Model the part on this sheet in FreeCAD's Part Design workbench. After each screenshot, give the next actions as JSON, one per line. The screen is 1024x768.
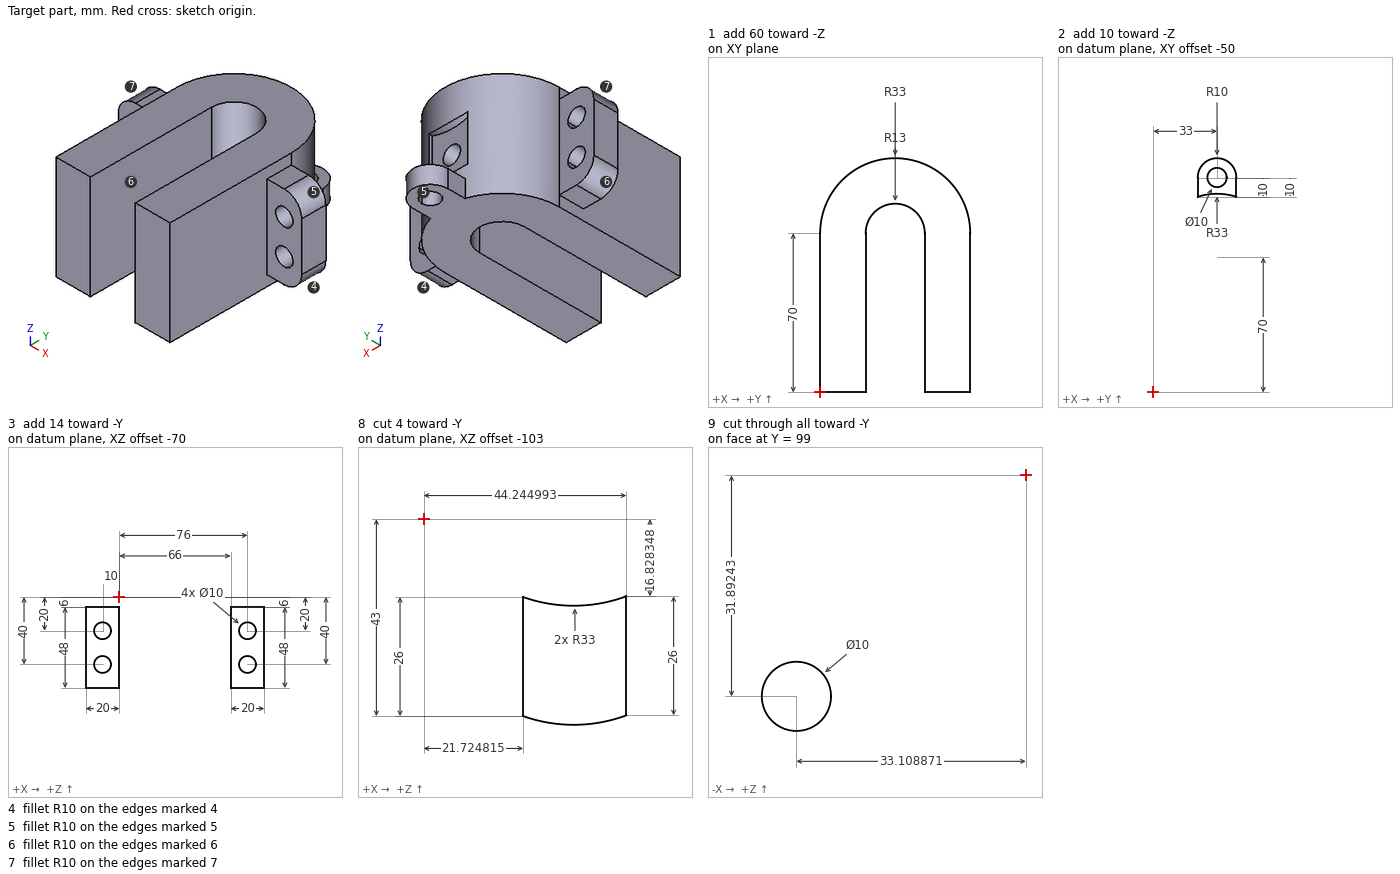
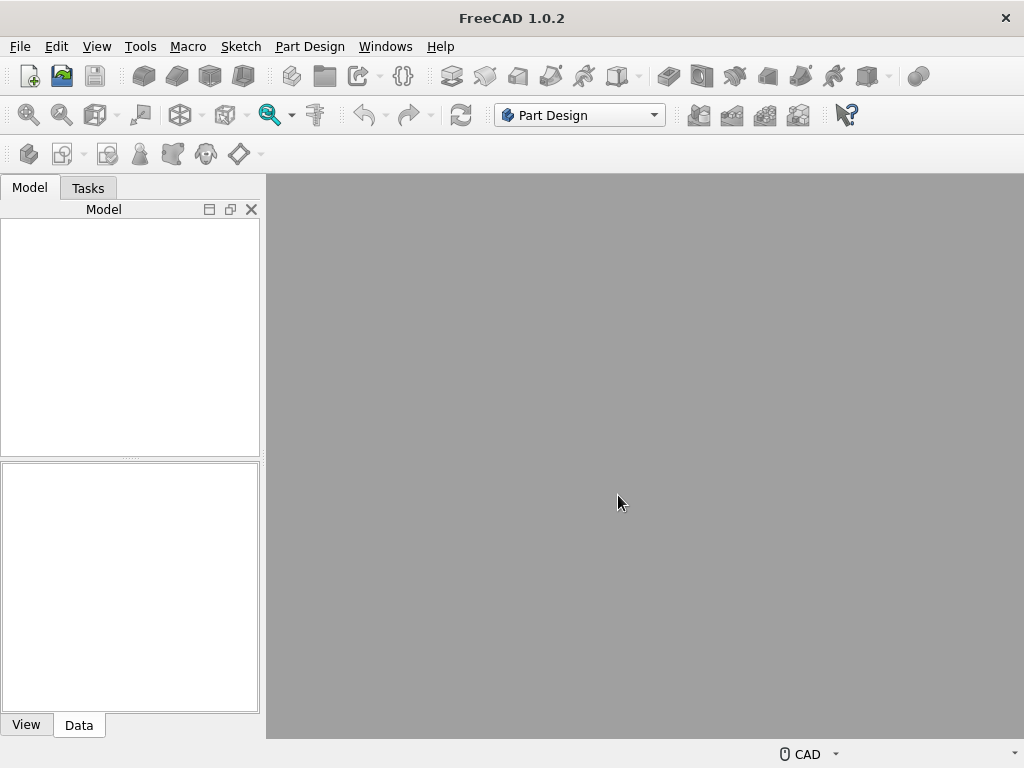
{"action": "left_click", "coordinate": [29, 76]}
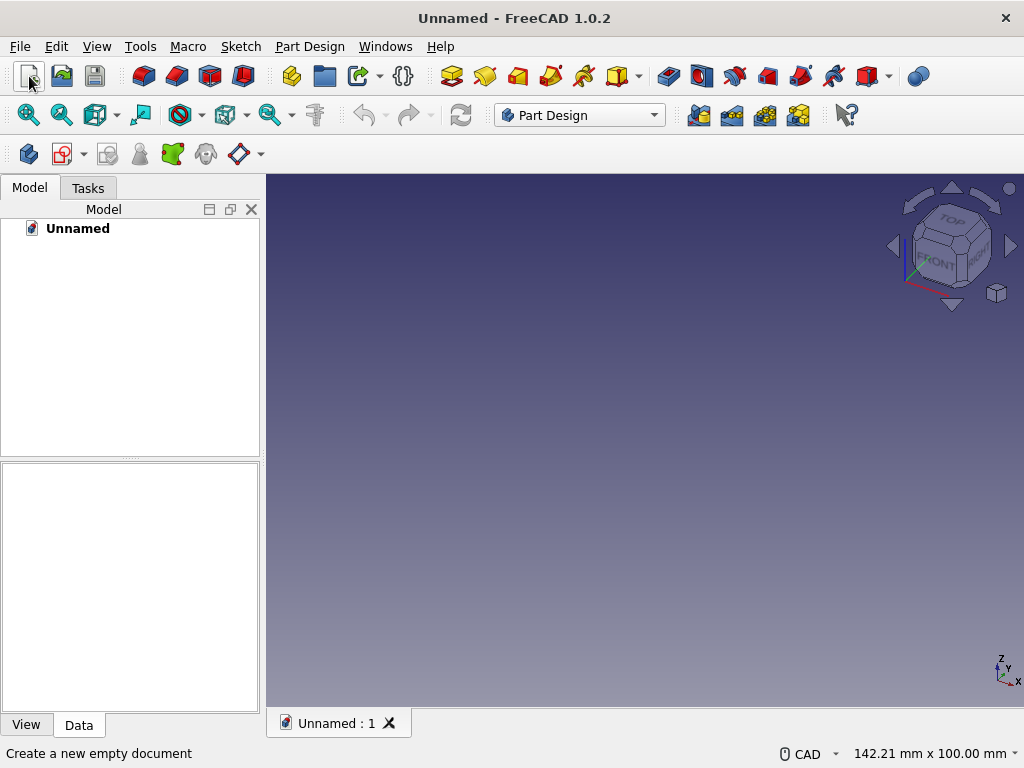
{"action": "left_click", "coordinate": [62, 154]}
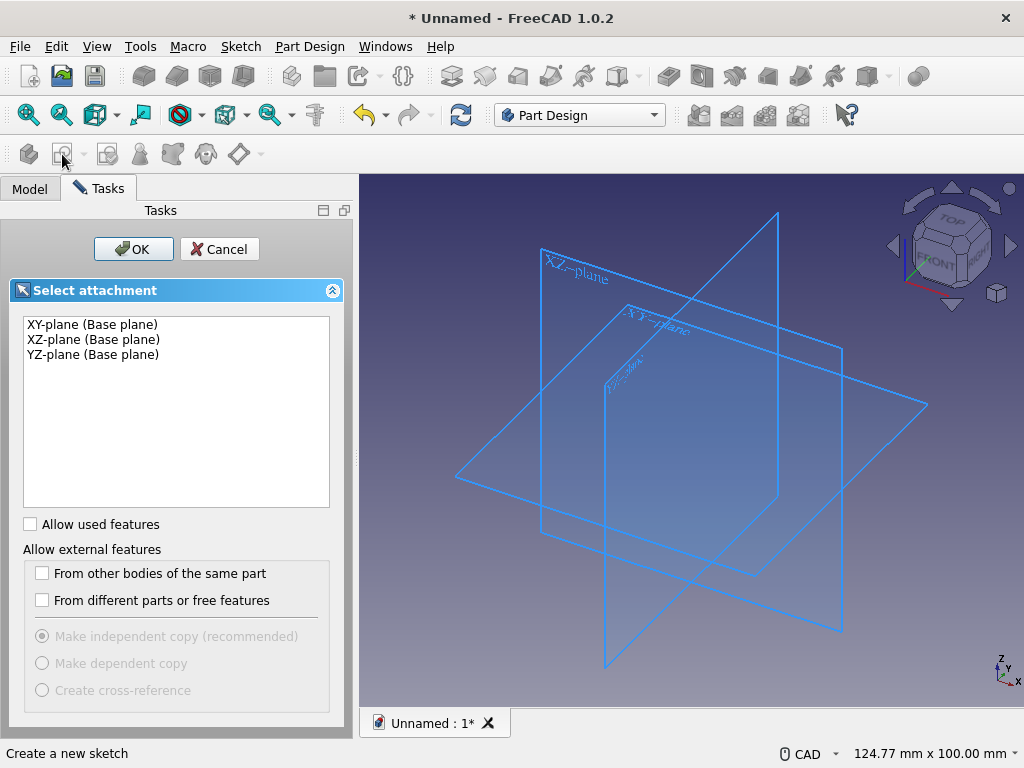
{"action": "left_click", "coordinate": [84, 324]}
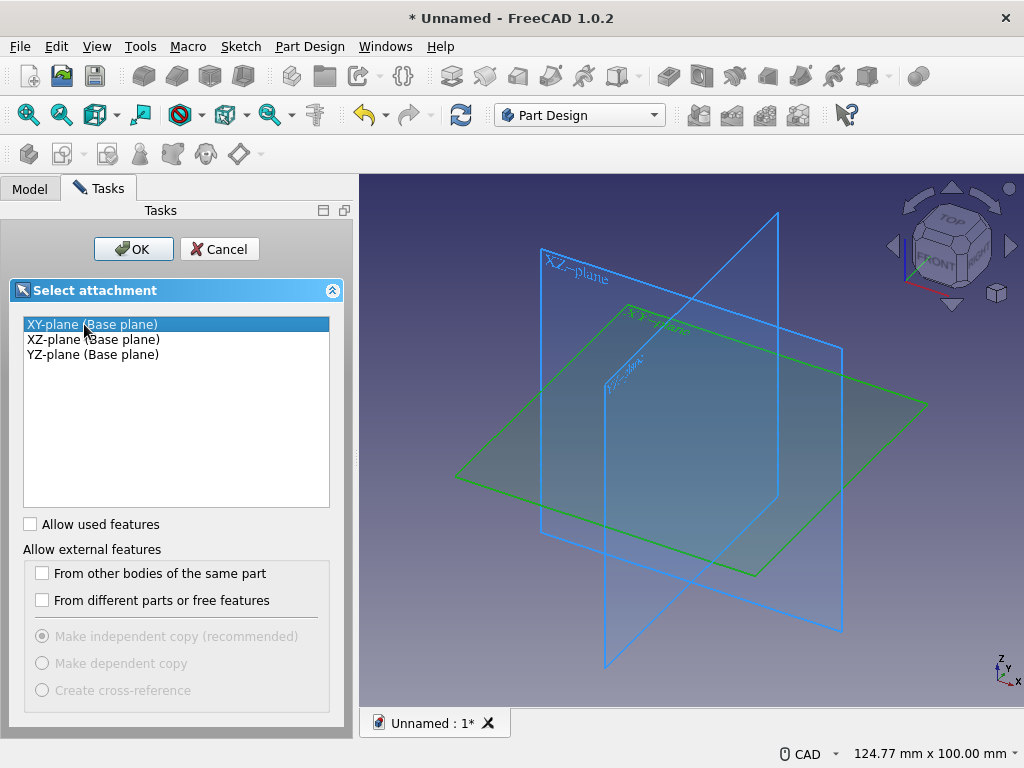
{"action": "left_click", "coordinate": [134, 249]}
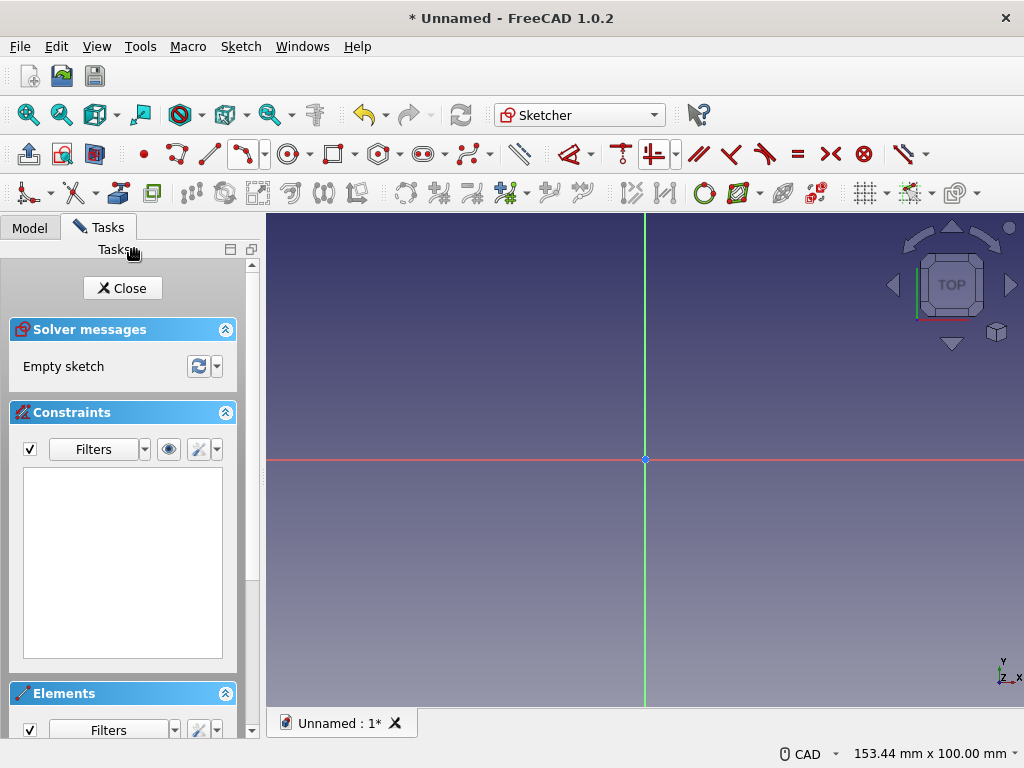
{"action": "scroll", "coordinate": [295, 679], "scroll_direction": "down", "scroll_amount": 3}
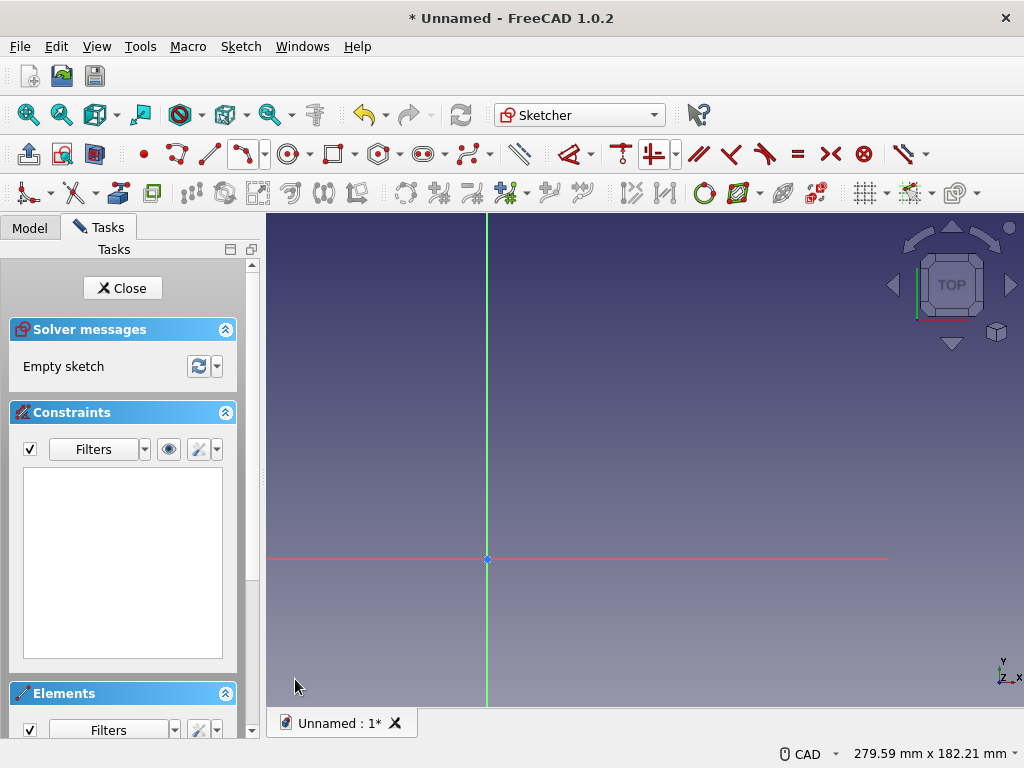
{"action": "key", "text": "g m"}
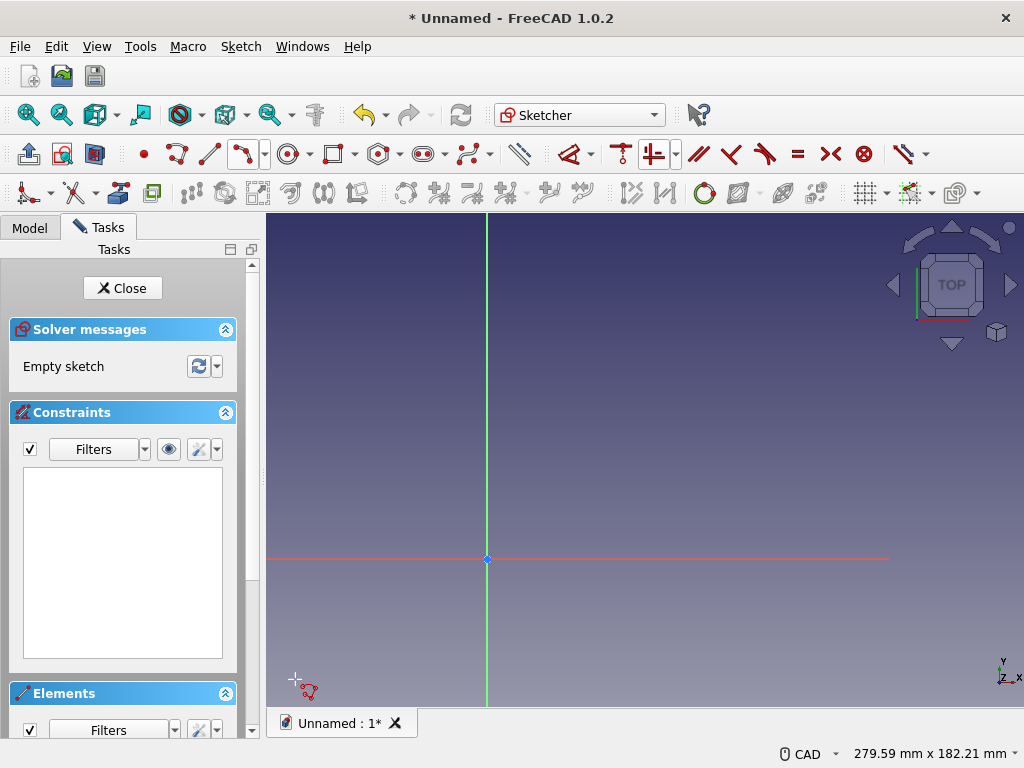
{"action": "left_click", "coordinate": [487, 369]}
{"action": "left_click", "coordinate": [487, 559]}
{"action": "left_click", "coordinate": [541, 550]}
{"action": "left_click", "coordinate": [541, 369]}
{"action": "right_click", "coordinate": [541, 369]}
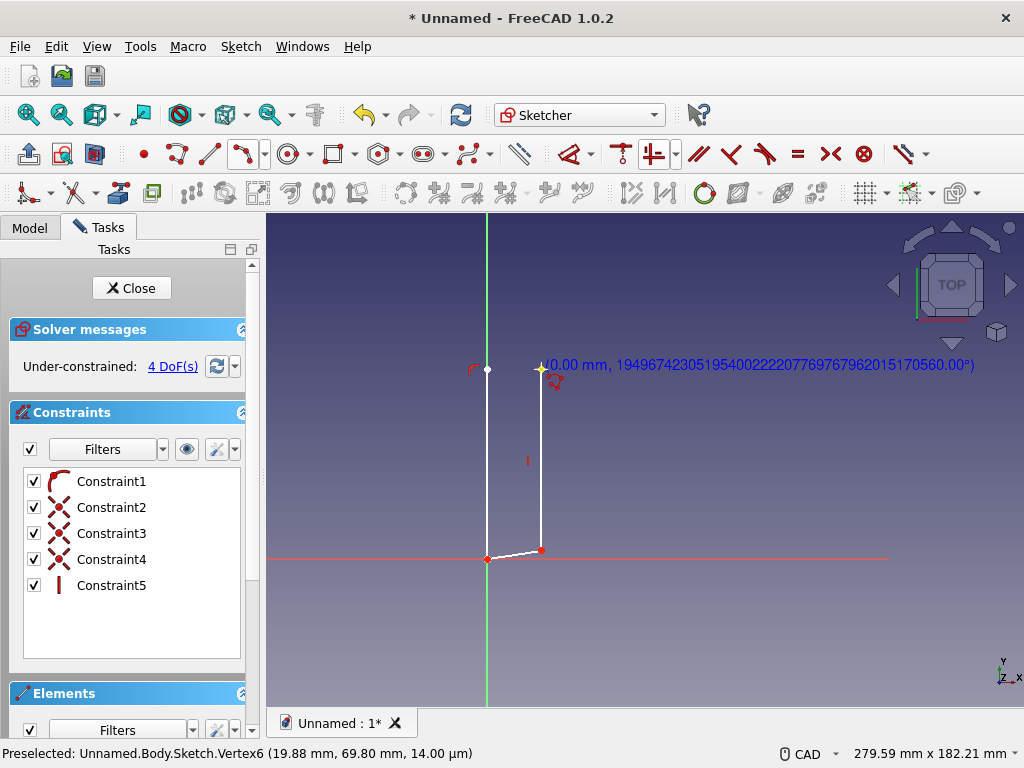
{"action": "left_click", "coordinate": [612, 369]}
{"action": "left_click", "coordinate": [612, 559]}
{"action": "left_click", "coordinate": [666, 550]}
{"action": "left_click", "coordinate": [666, 369]}
{"action": "right_click", "coordinate": [666, 369]}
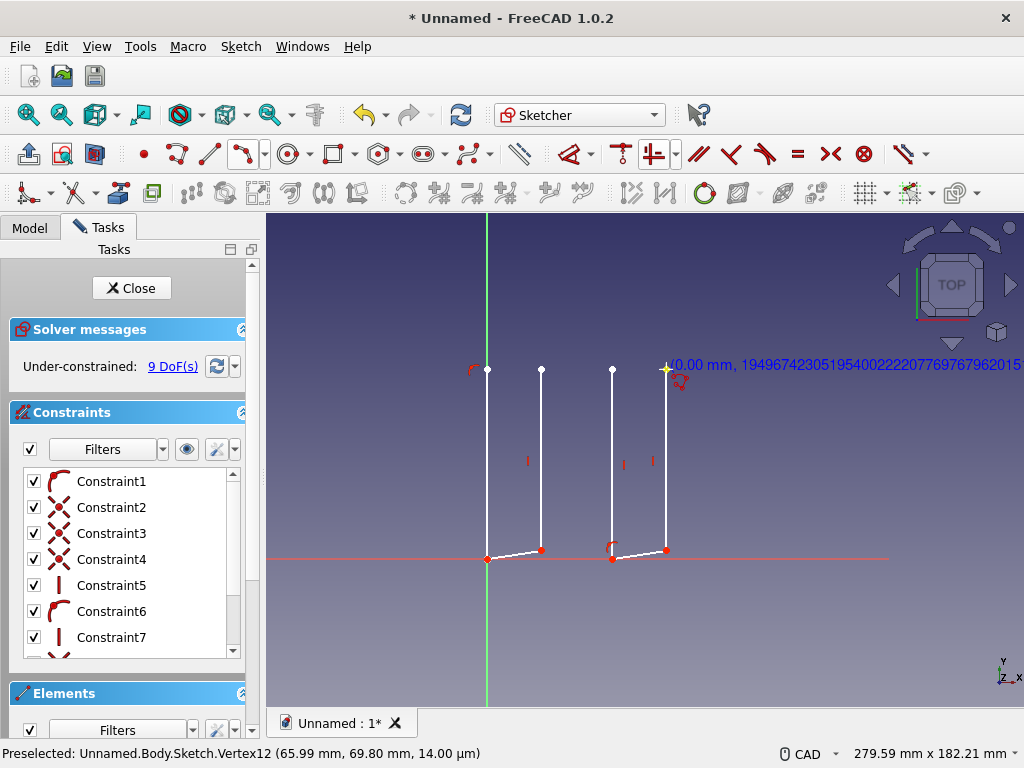
{"action": "left_click", "coordinate": [242, 154]}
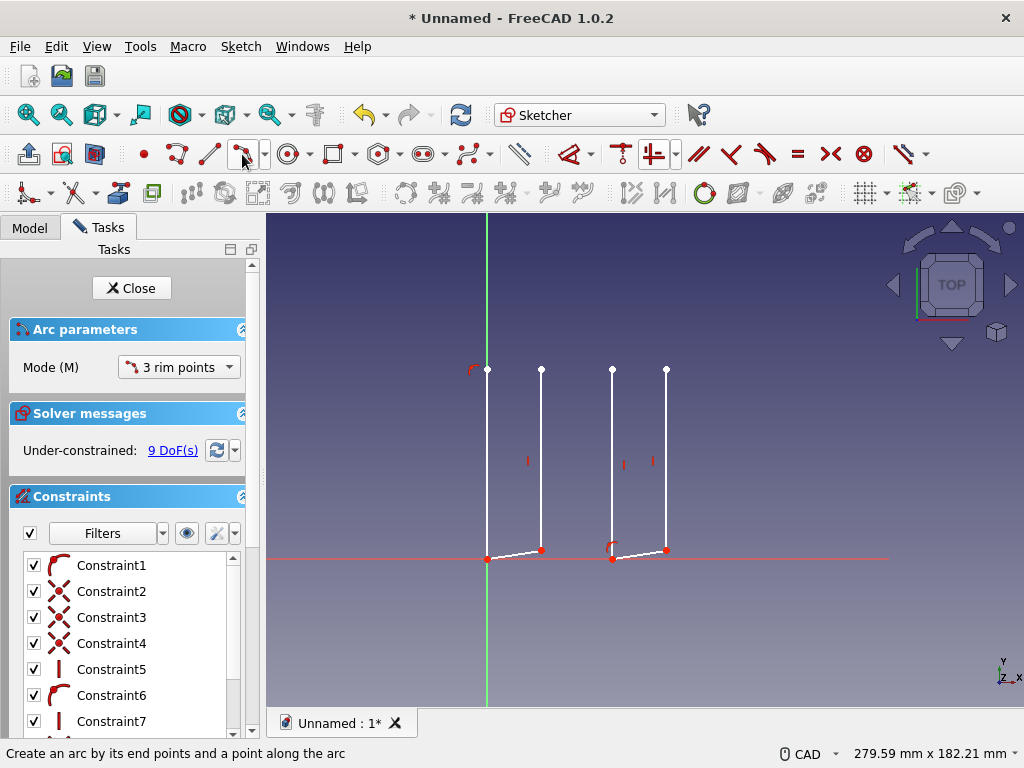
{"action": "left_click", "coordinate": [541, 370]}
{"action": "left_click", "coordinate": [612, 370]}
{"action": "left_click", "coordinate": [577, 334]}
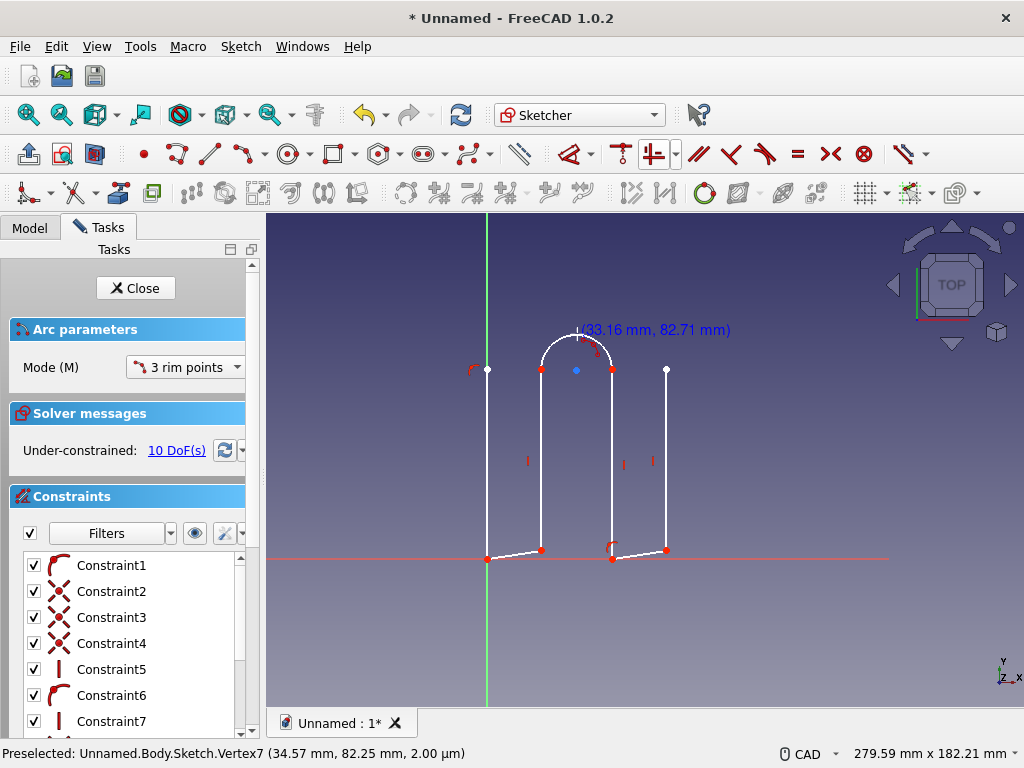
{"action": "left_click", "coordinate": [666, 370]}
{"action": "left_click", "coordinate": [487, 370]}
{"action": "left_click", "coordinate": [577, 280]}
{"action": "key", "text": "Escape"}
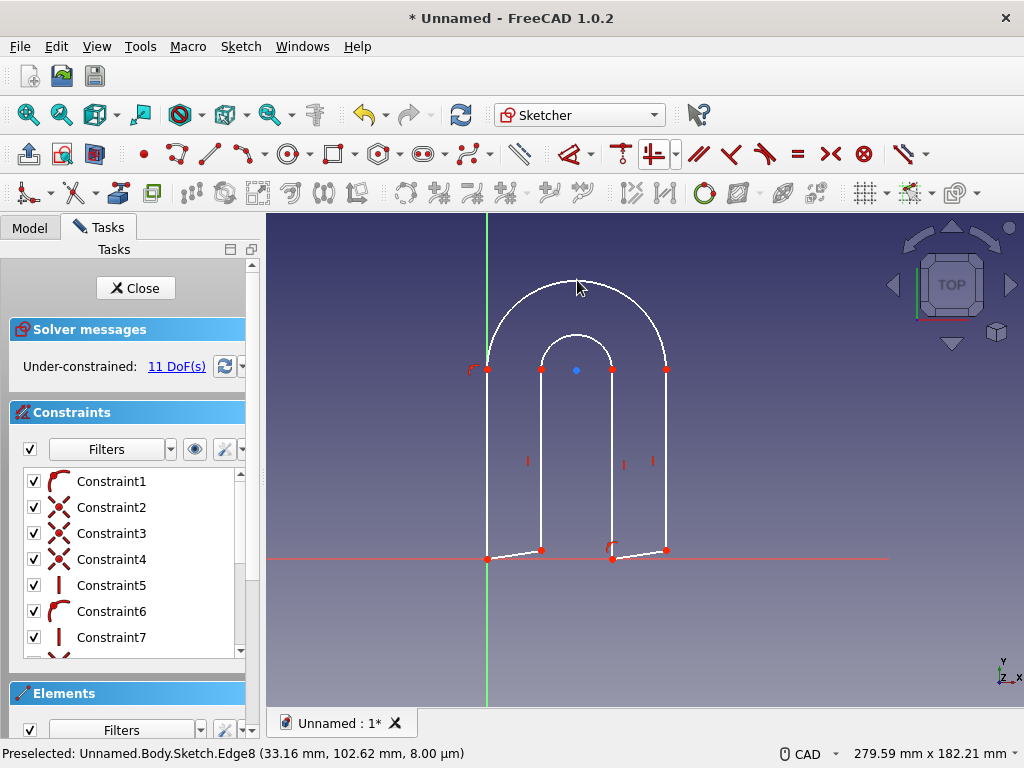
{"action": "left_click", "coordinate": [487, 427]}